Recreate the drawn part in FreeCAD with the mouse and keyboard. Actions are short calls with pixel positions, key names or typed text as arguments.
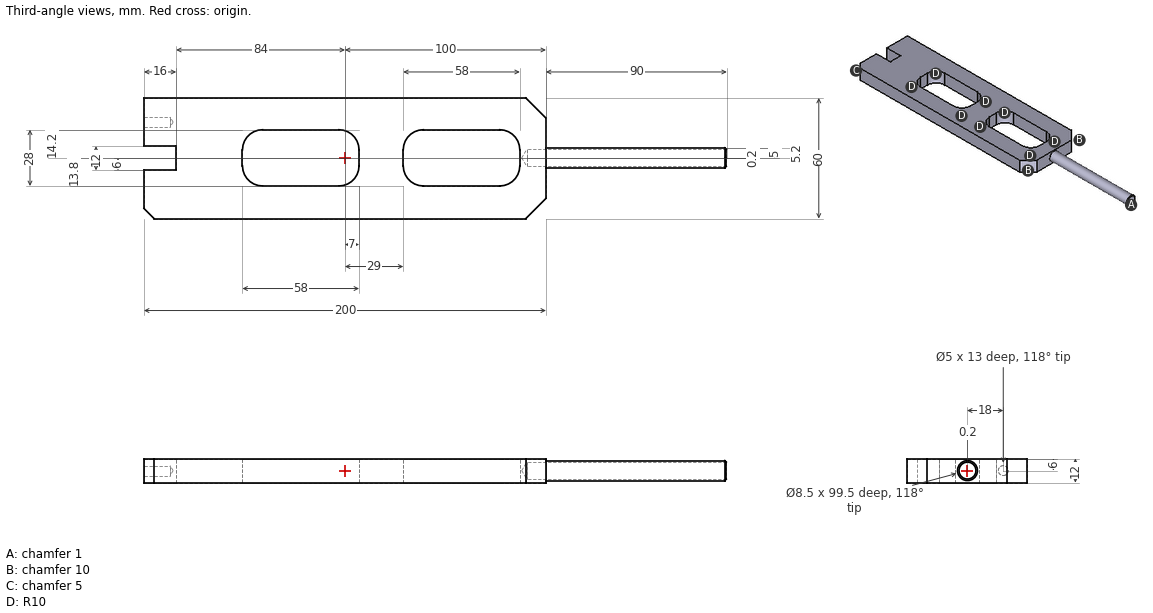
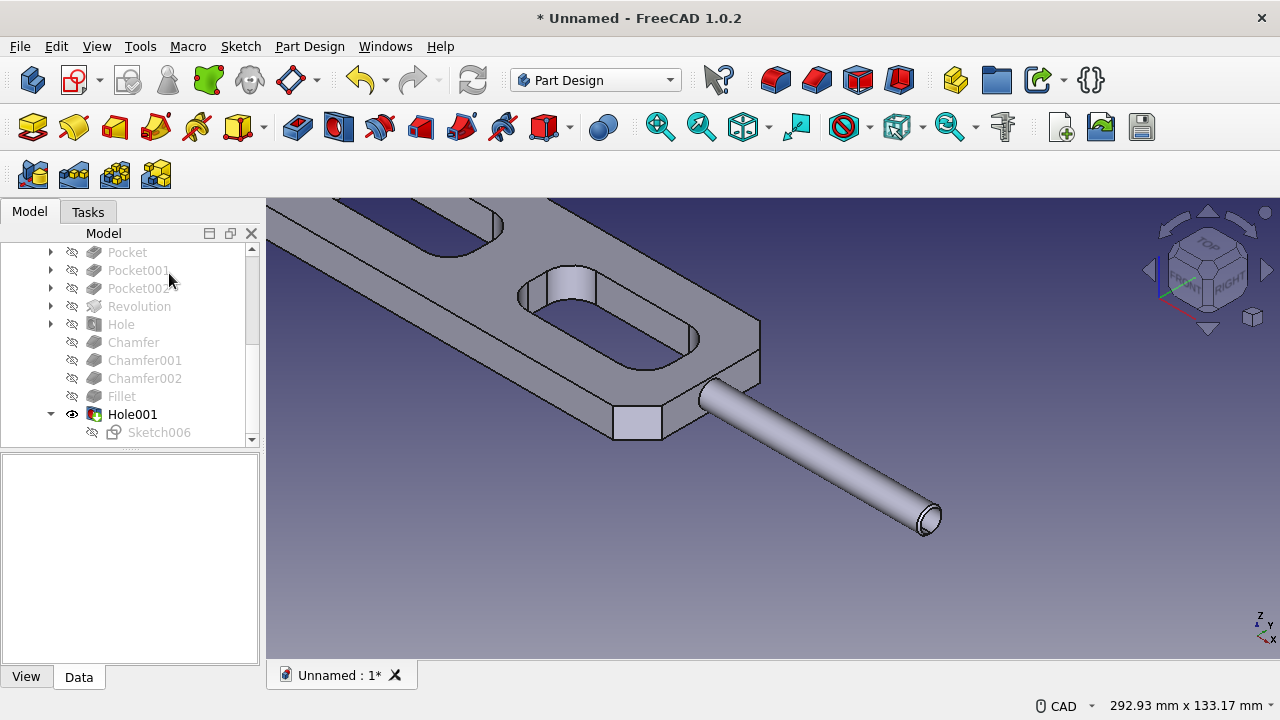
key(v)
key(f)